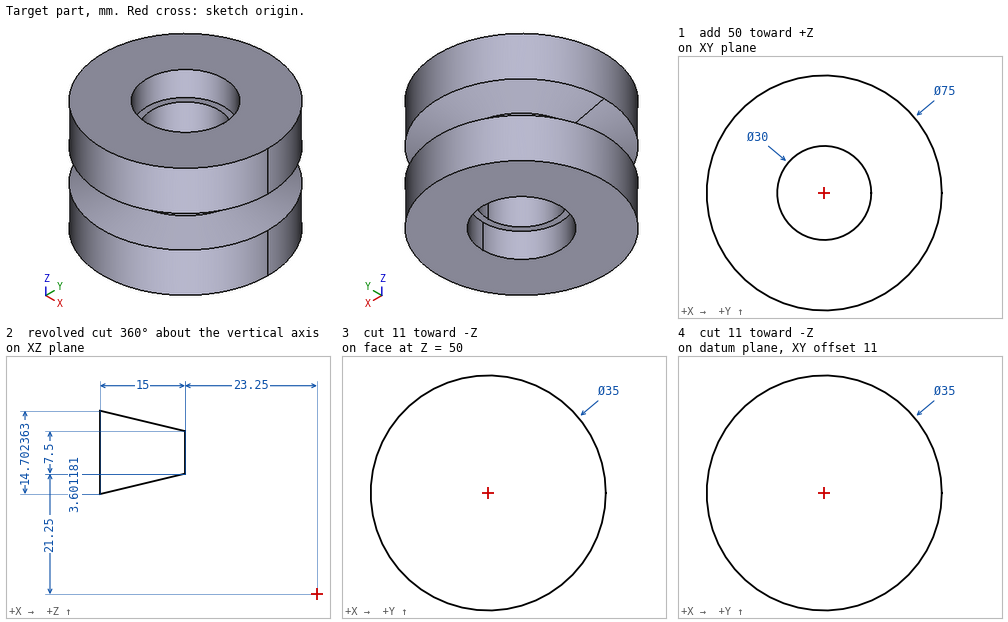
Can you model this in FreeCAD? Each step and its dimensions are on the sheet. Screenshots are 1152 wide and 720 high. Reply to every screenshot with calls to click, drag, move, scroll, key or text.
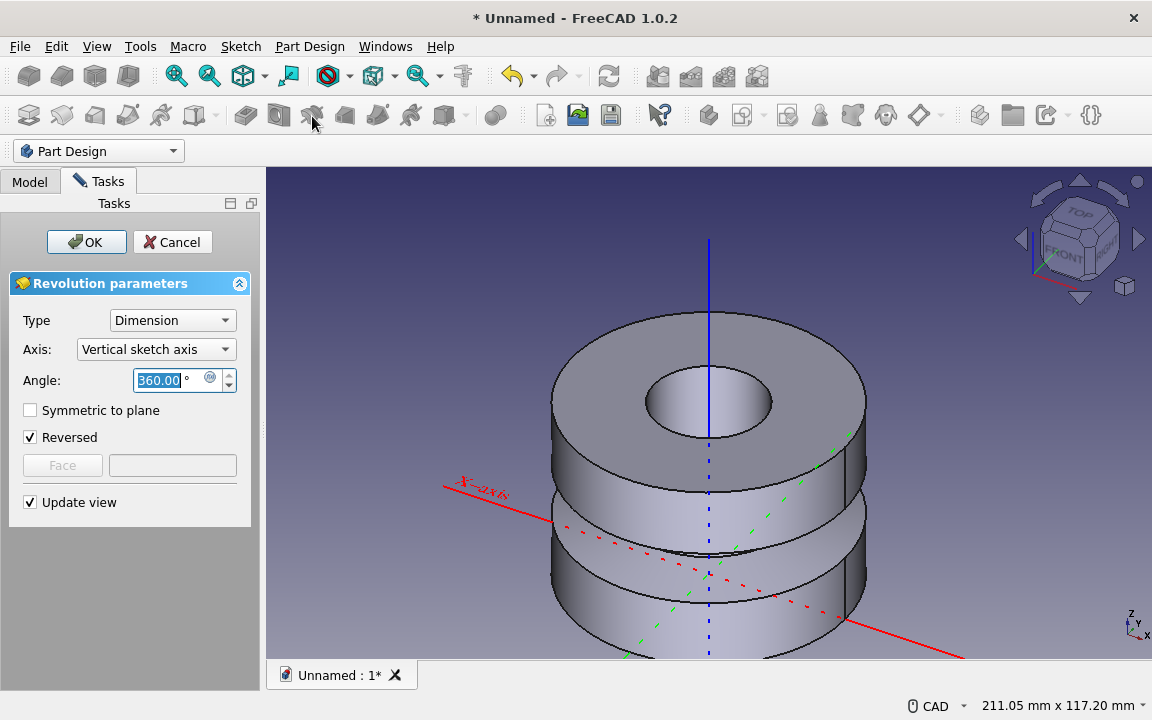
click(87, 242)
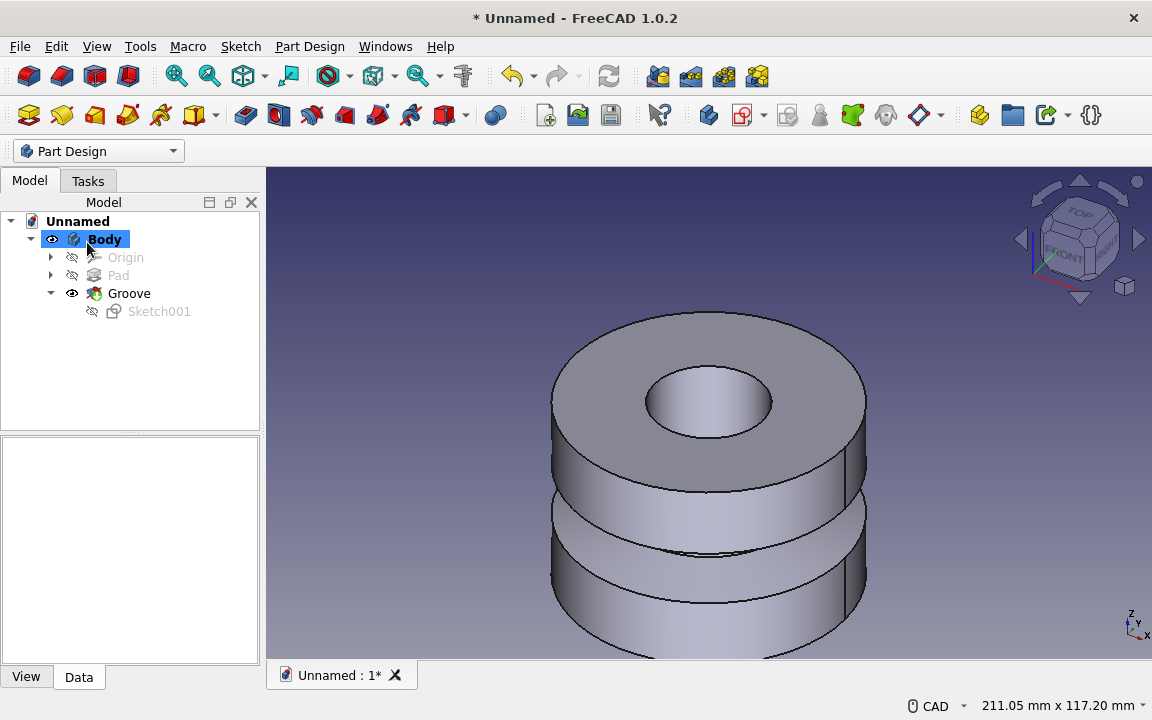
click(177, 76)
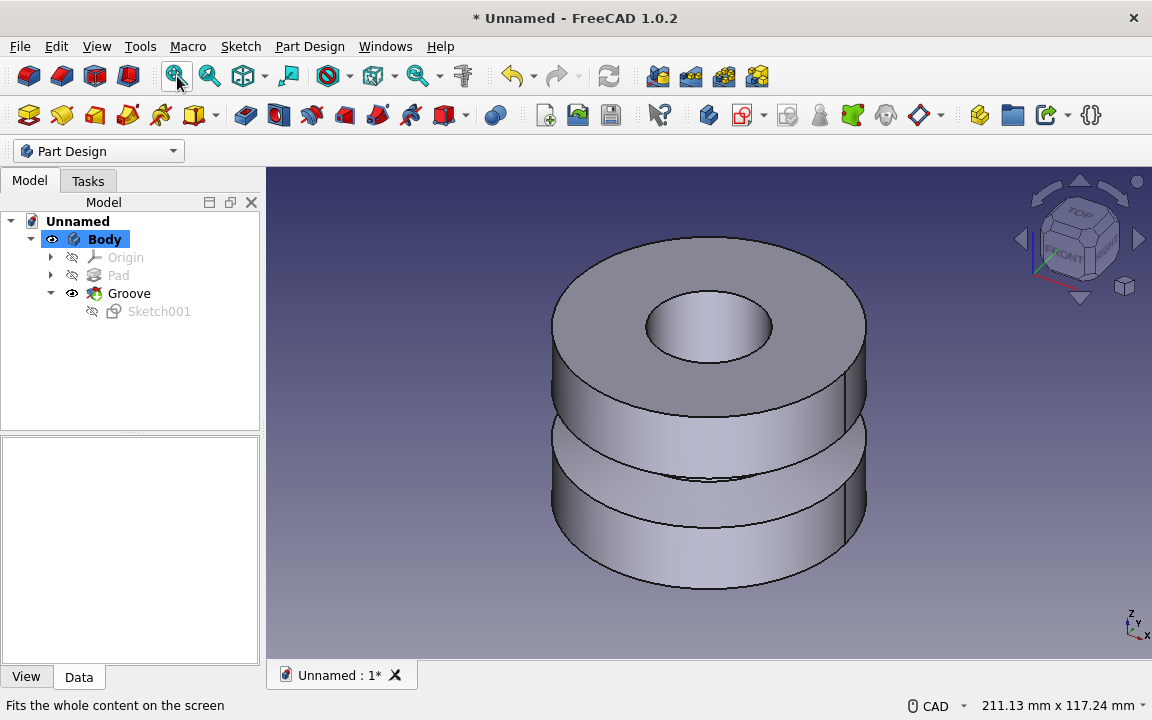
click(715, 268)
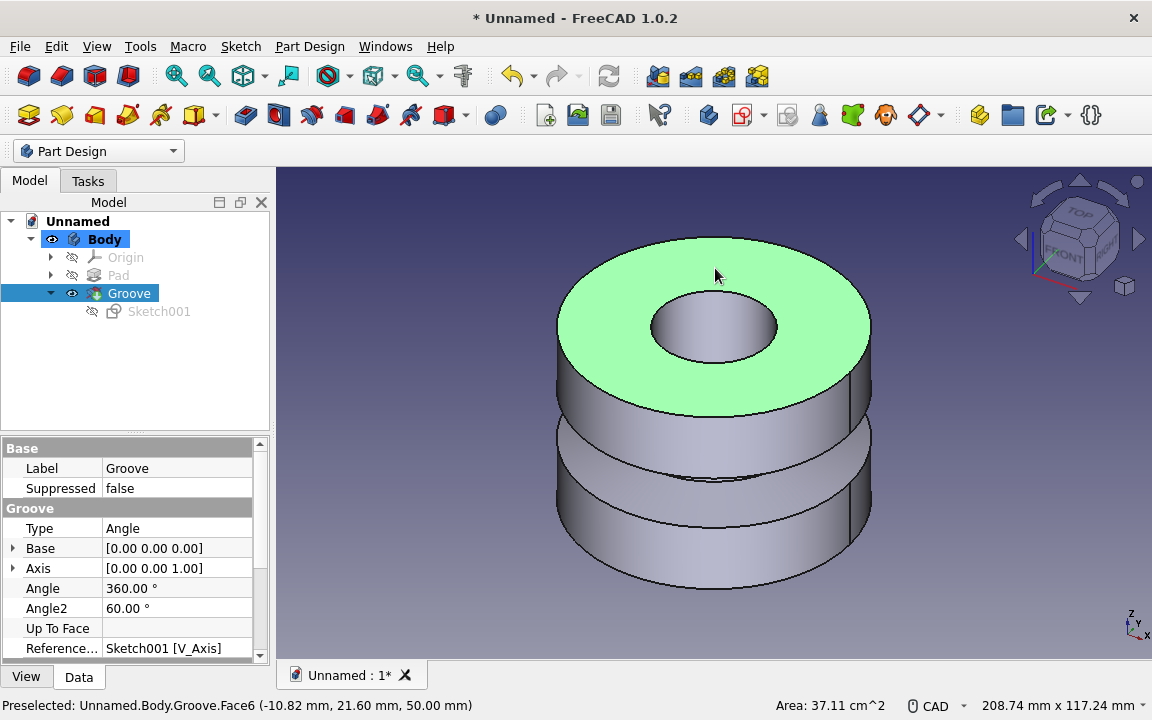
click(742, 116)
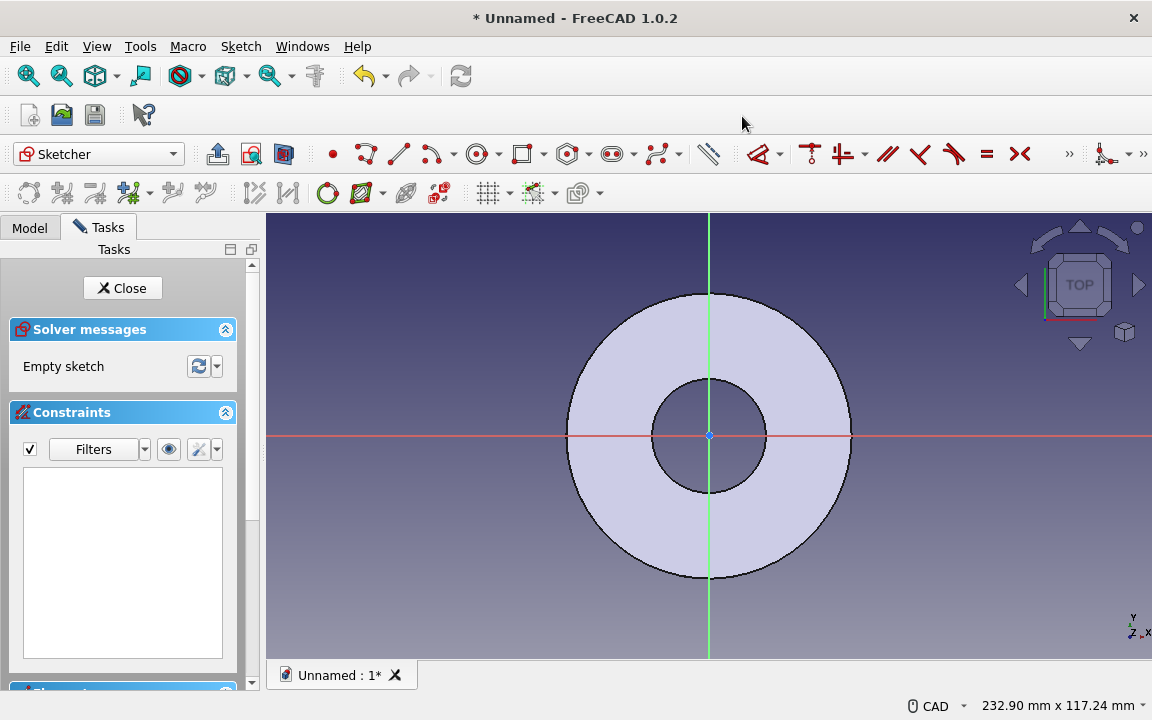
scroll(765, 436, up, 4)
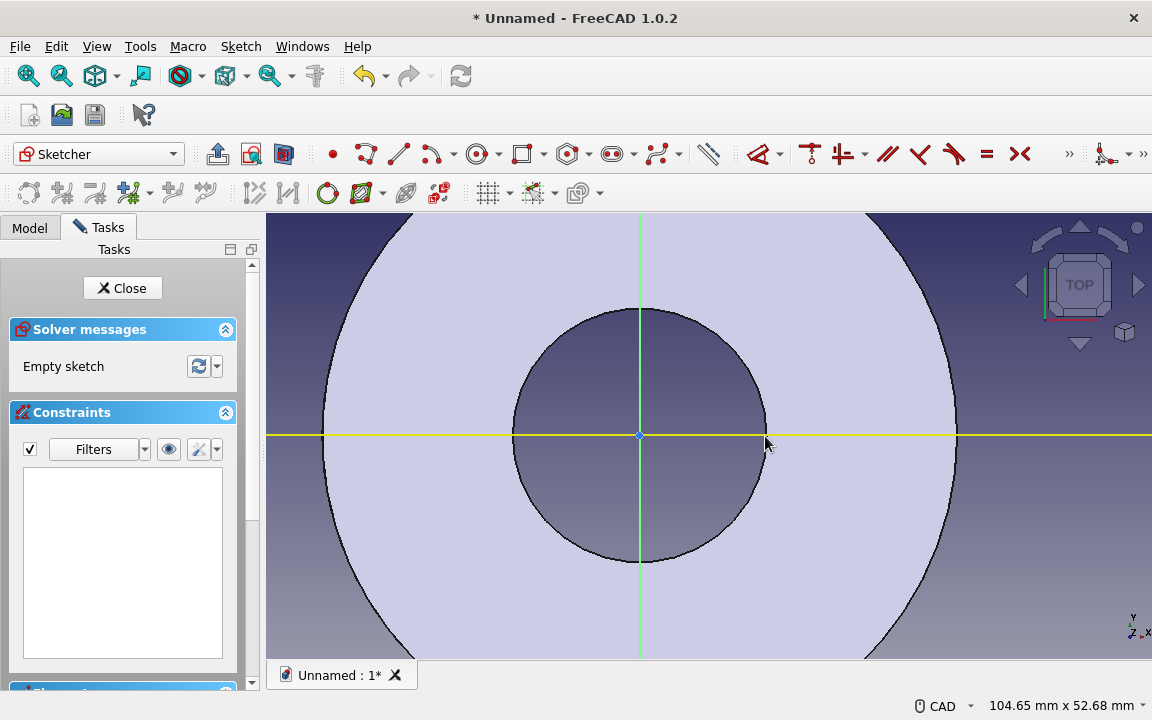
key(g)
key(c)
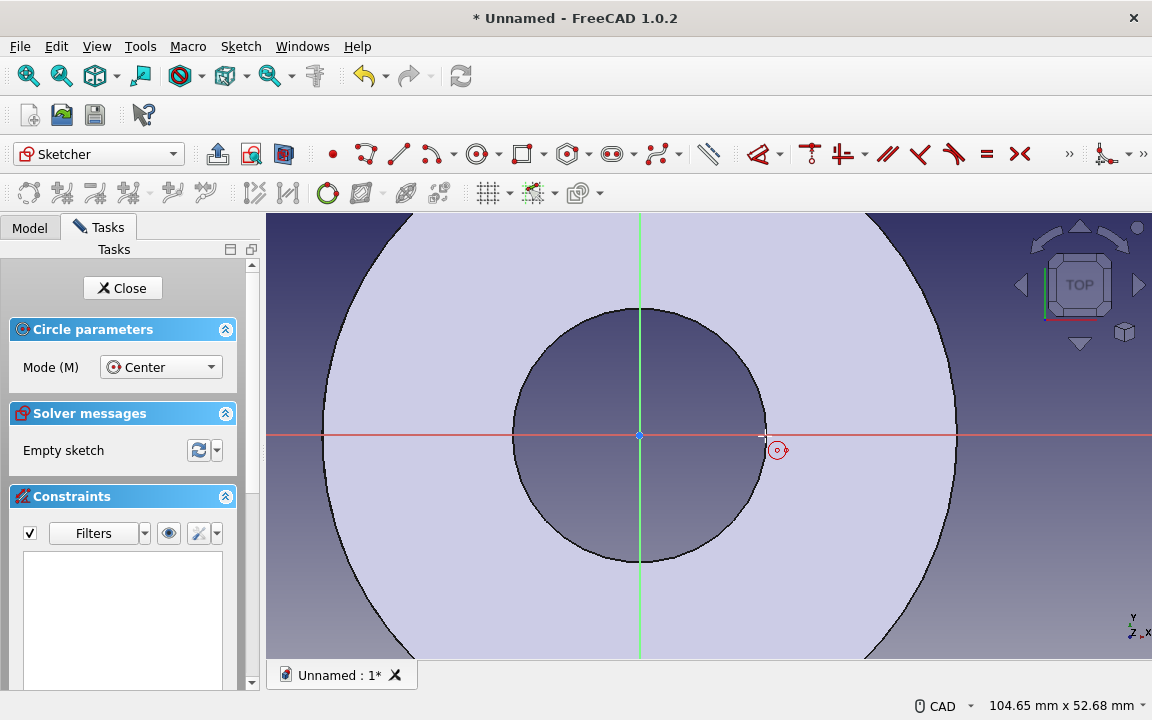
click(640, 435)
move(744, 331)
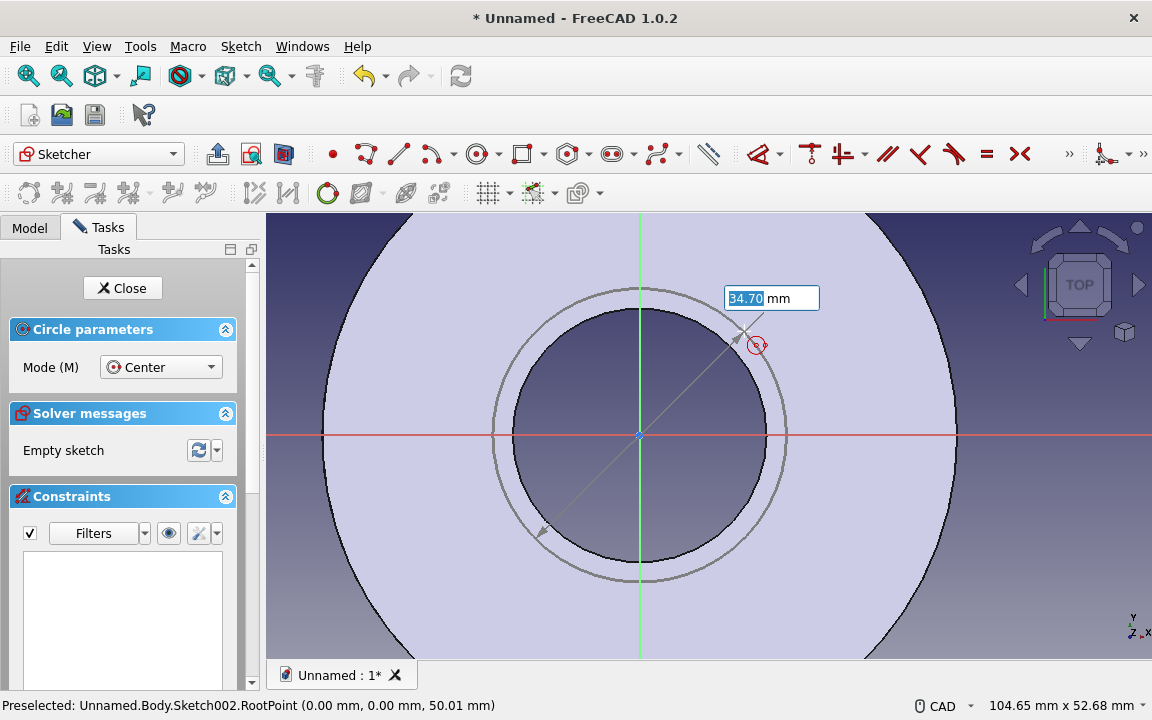
text(35)
key(Return)
key(Escape)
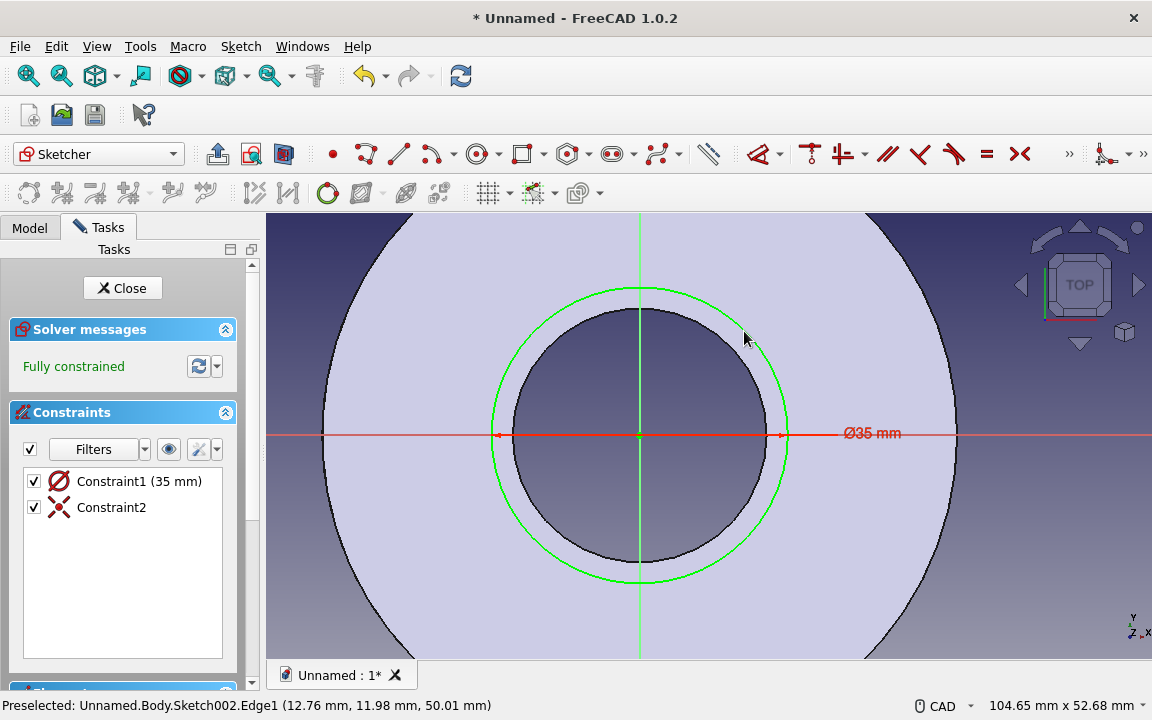
click(123, 288)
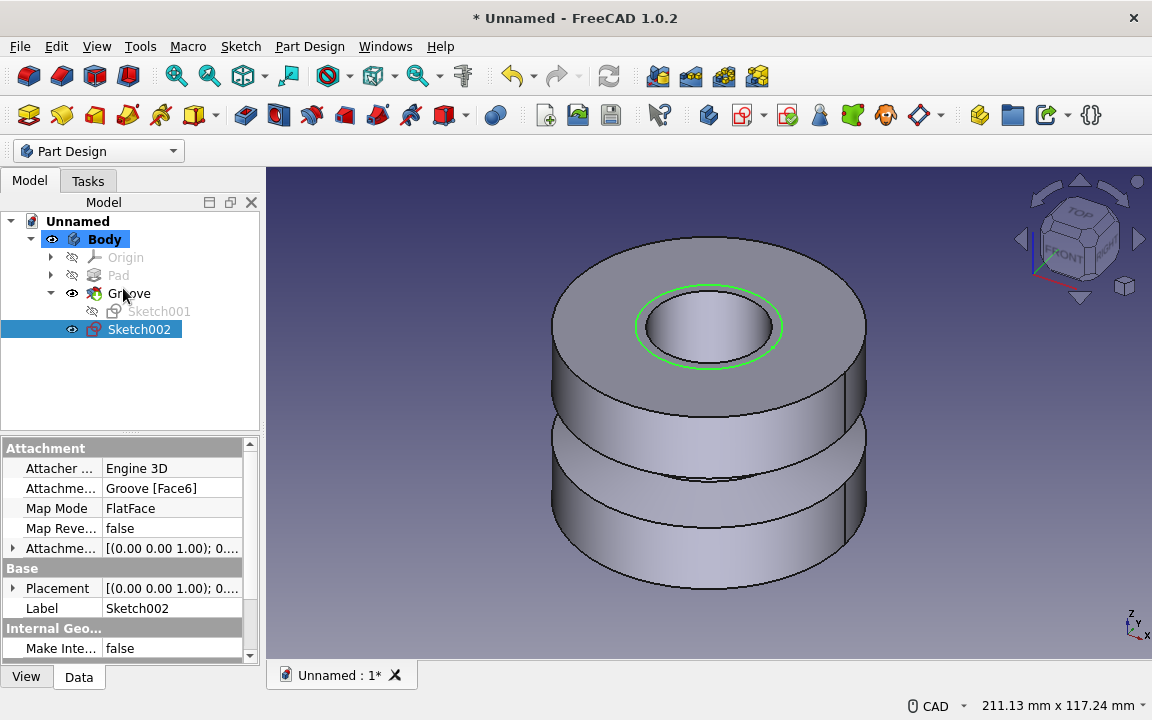
click(246, 116)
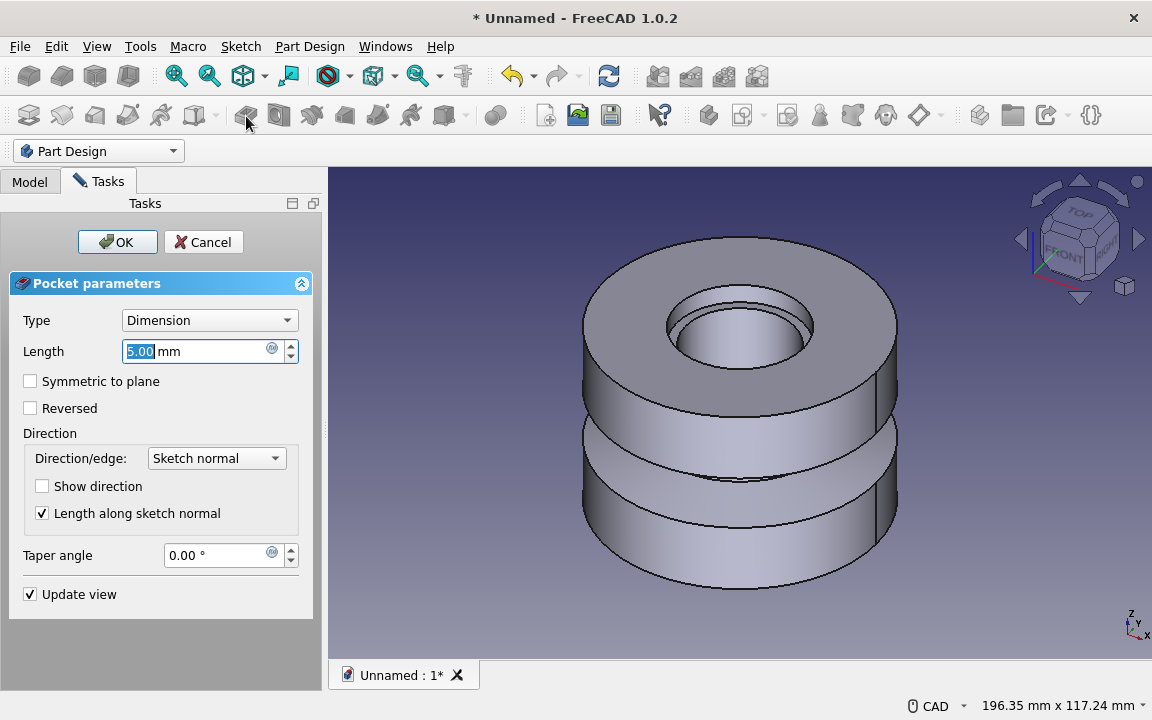
text(11)
key(Tab)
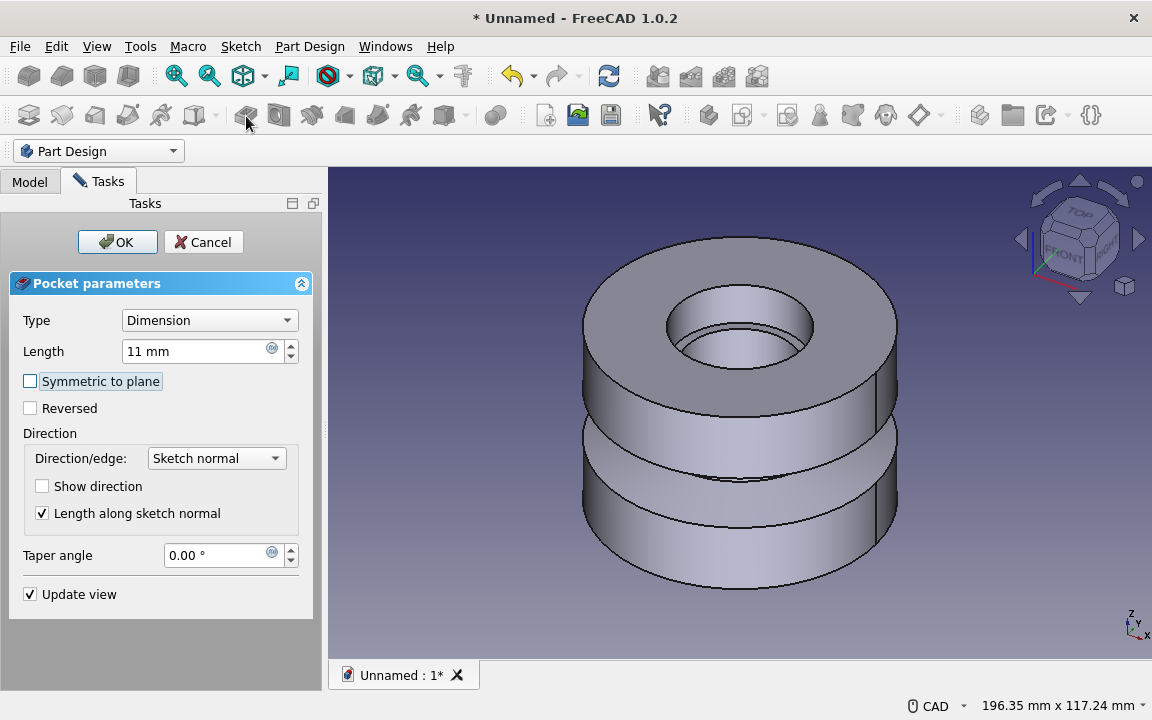
click(118, 242)